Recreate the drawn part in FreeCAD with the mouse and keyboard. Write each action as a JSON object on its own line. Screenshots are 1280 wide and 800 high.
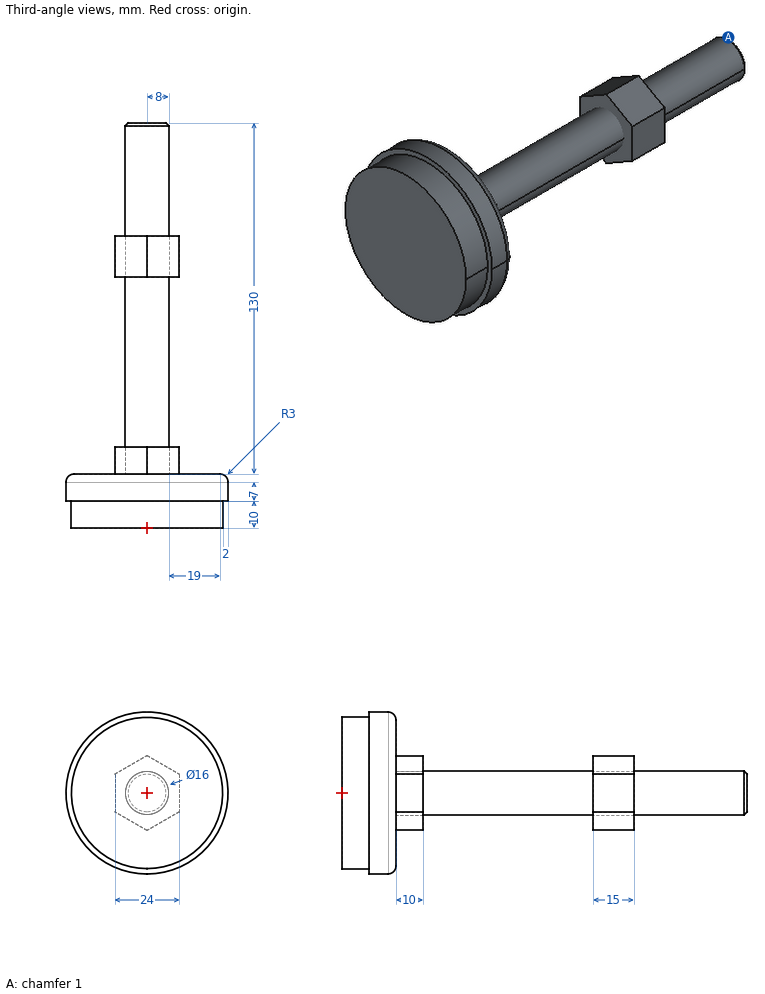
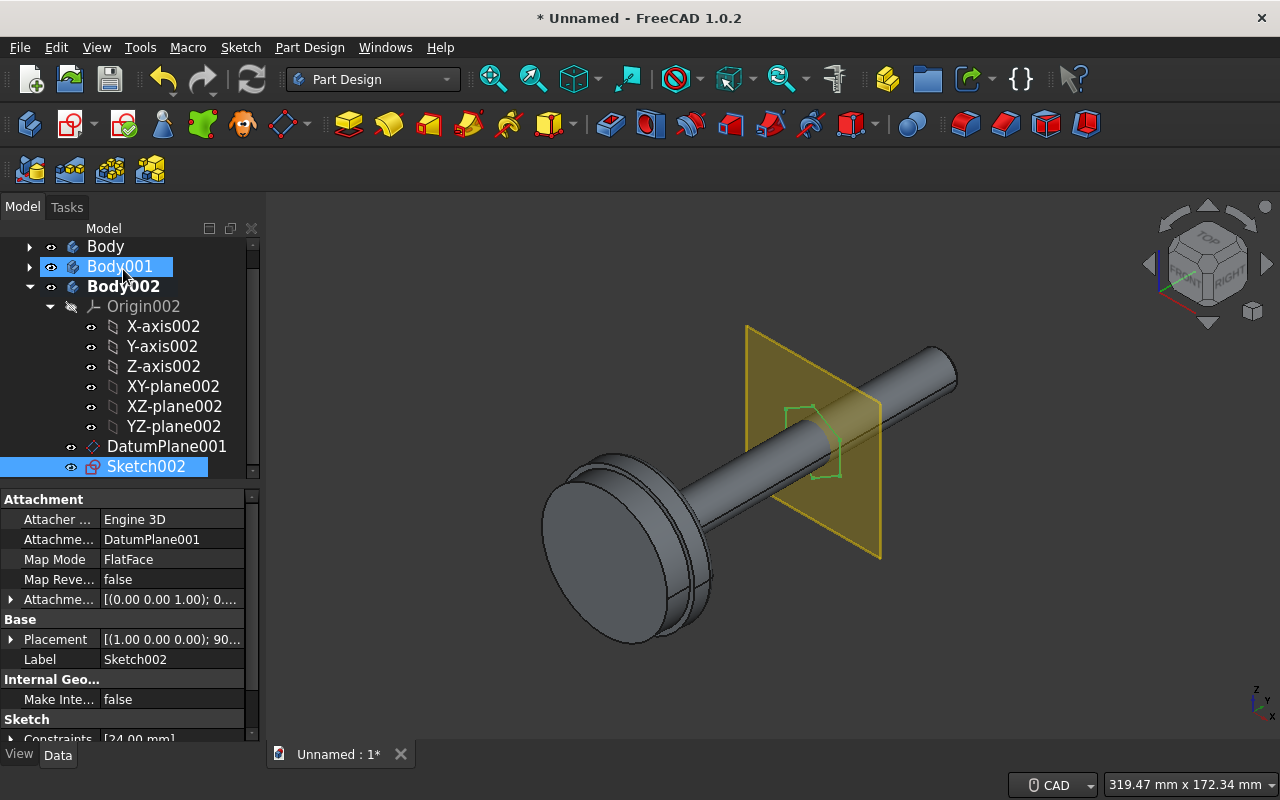
{"action": "left_click", "coordinate": [350, 124]}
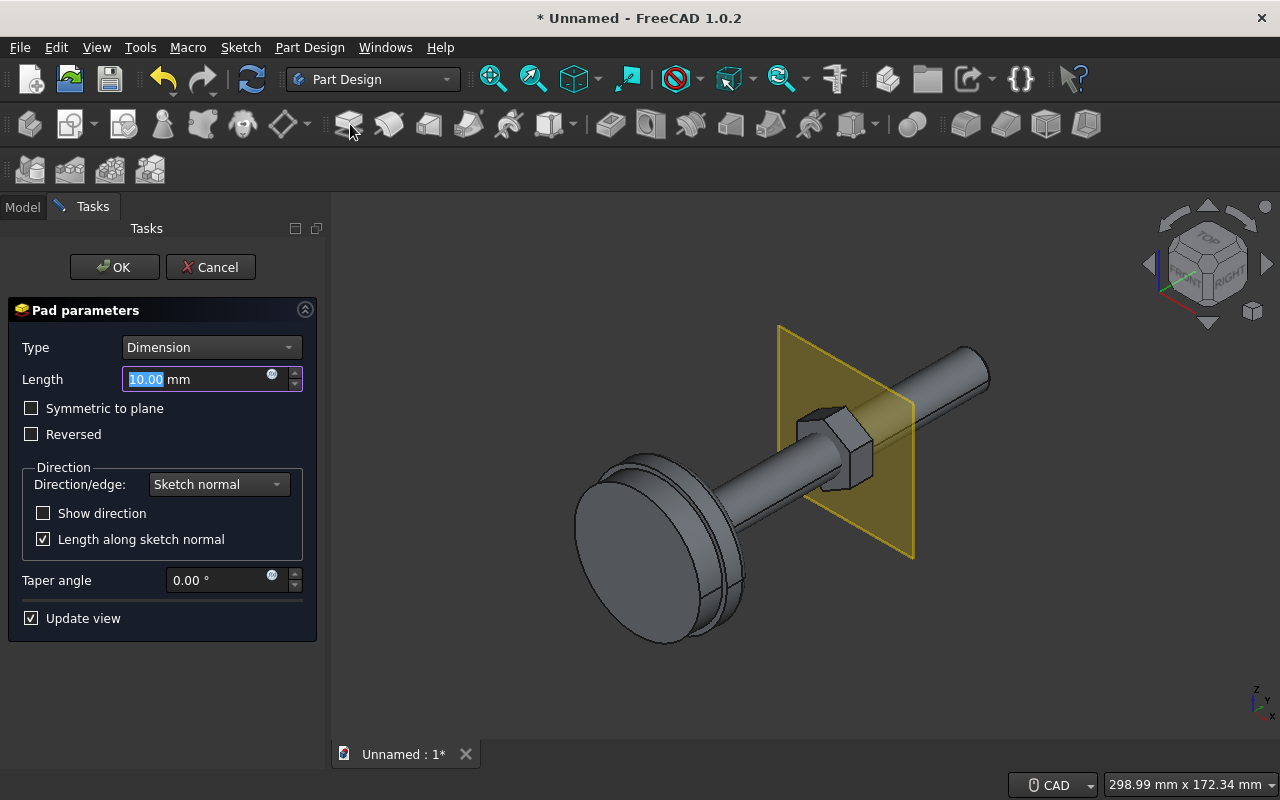
{"action": "type", "text": "15"}
{"action": "key", "text": "Tab"}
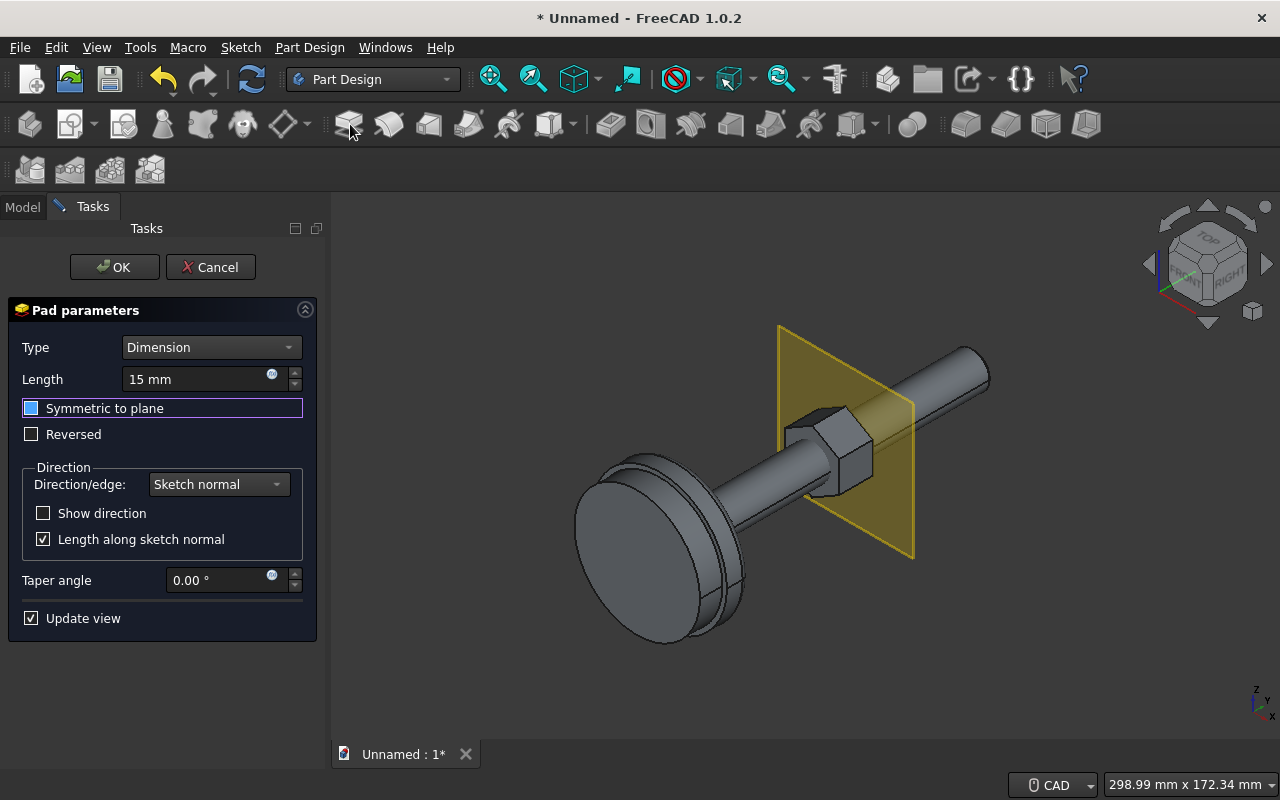
{"action": "left_click", "coordinate": [30, 434]}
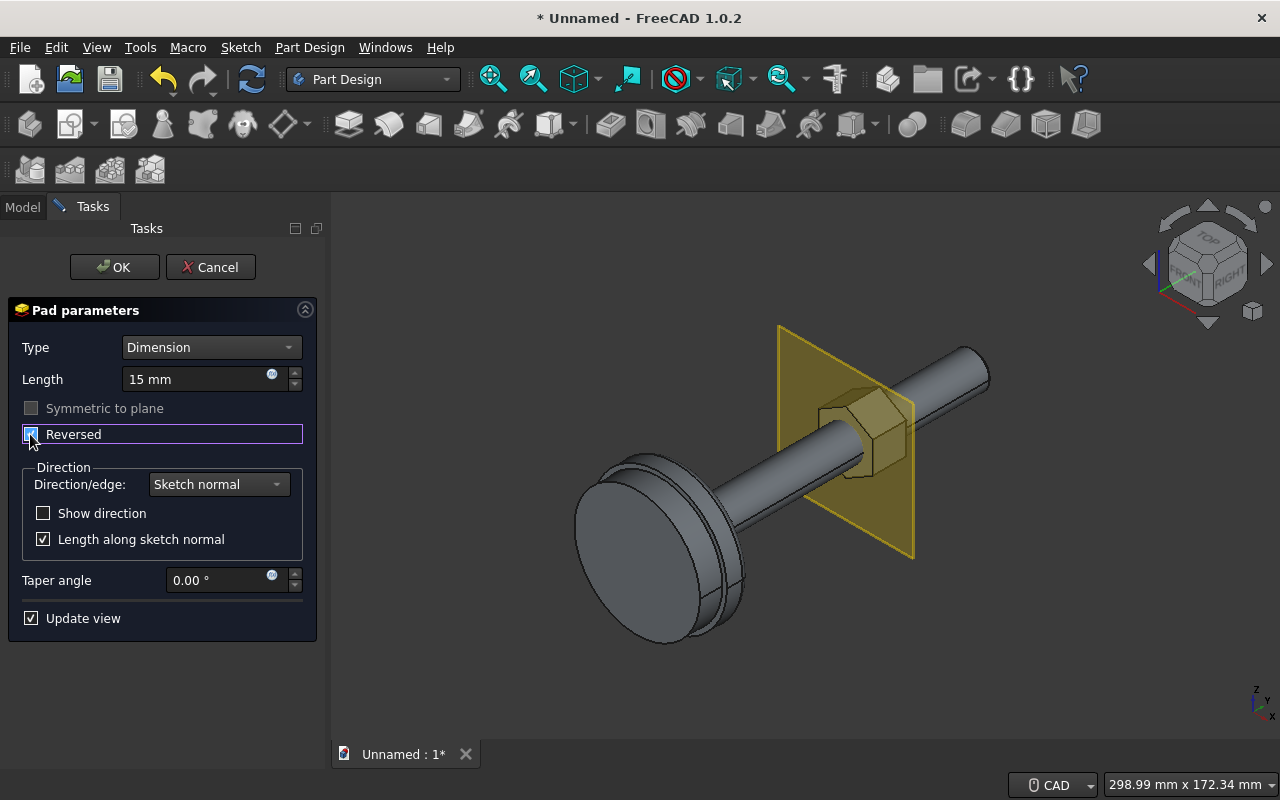
{"action": "left_click", "coordinate": [115, 267]}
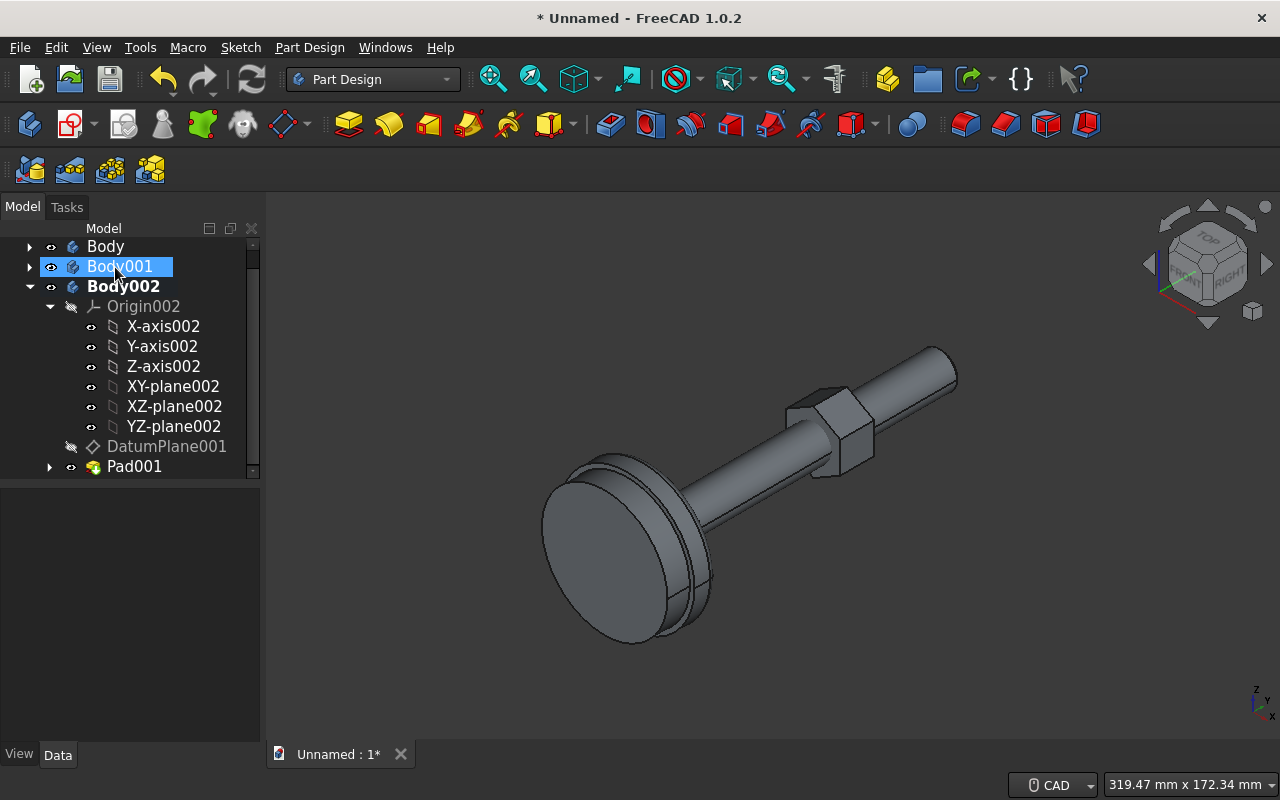
{"action": "left_click", "coordinate": [494, 80]}